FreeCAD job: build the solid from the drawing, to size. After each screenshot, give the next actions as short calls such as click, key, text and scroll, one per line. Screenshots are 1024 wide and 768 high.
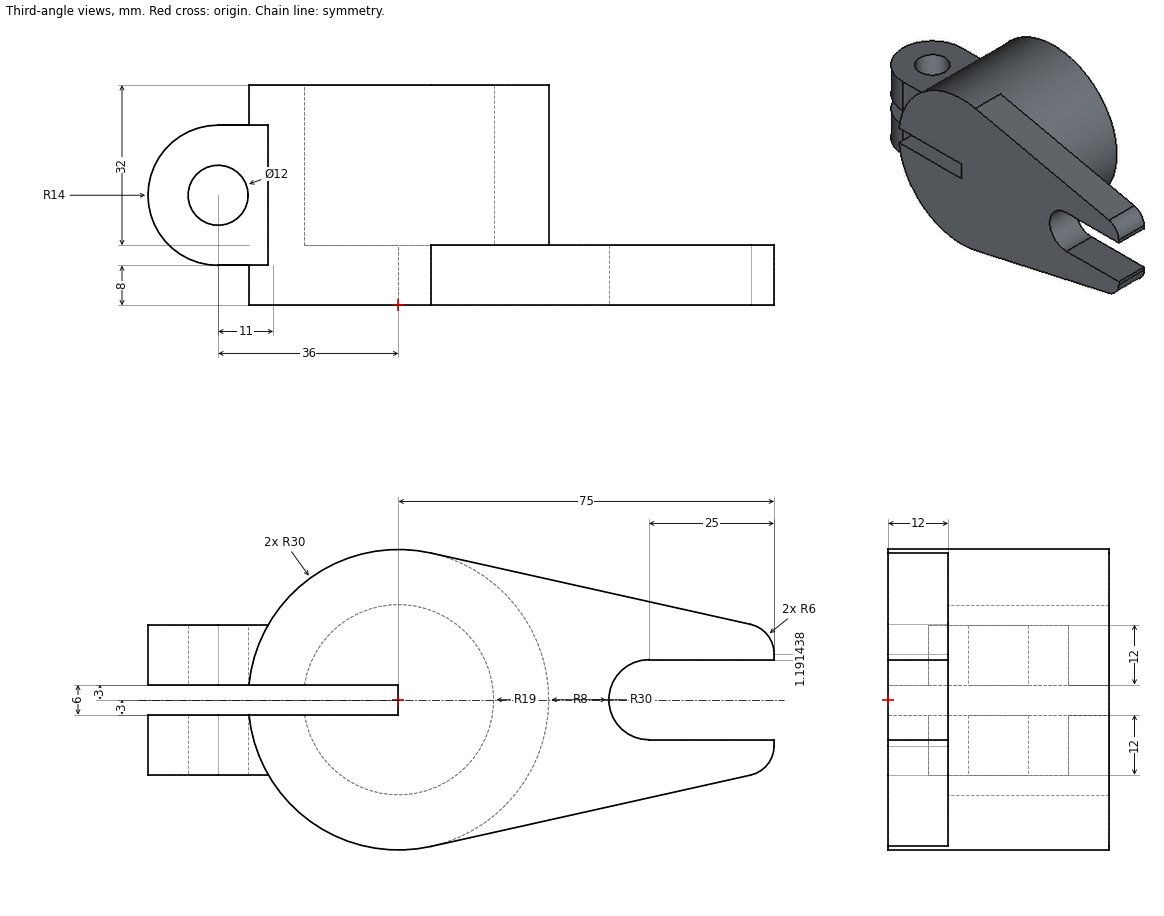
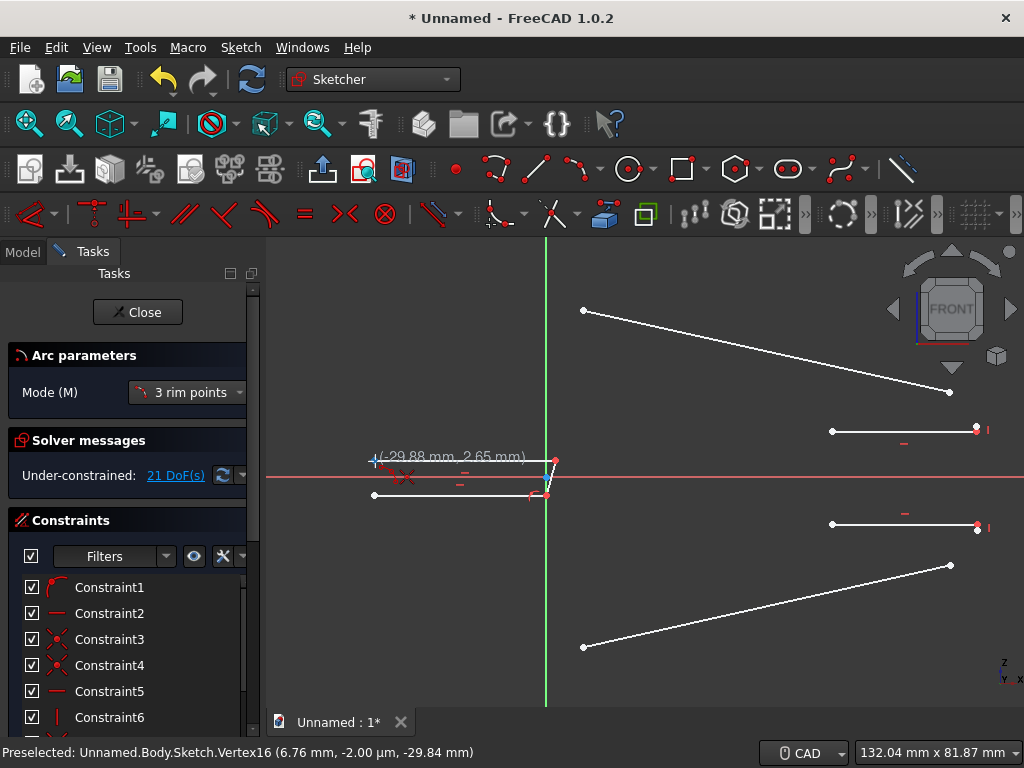
click(375, 461)
click(584, 311)
click(446, 338)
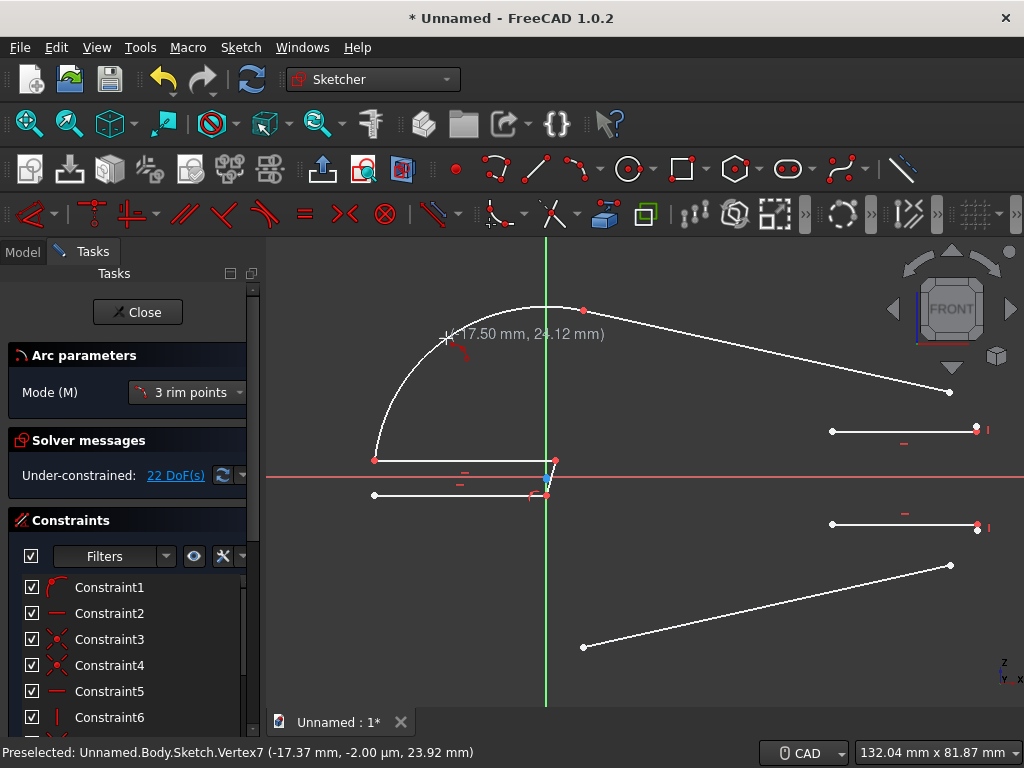
scroll(374, 461, down, 2)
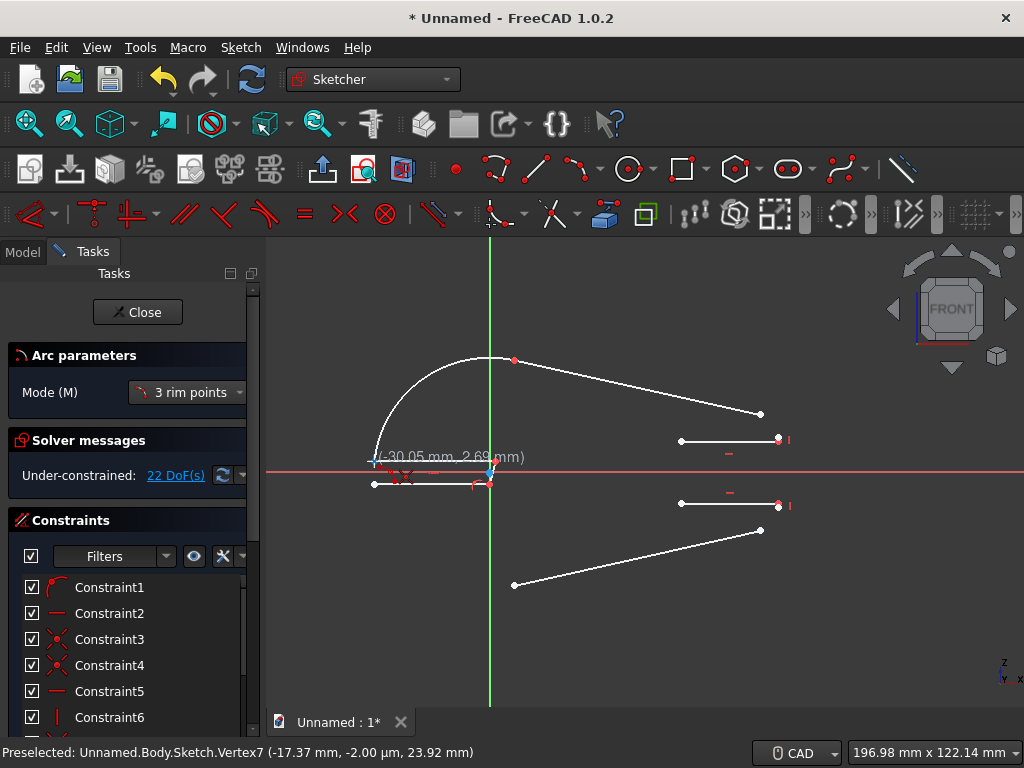
click(760, 415)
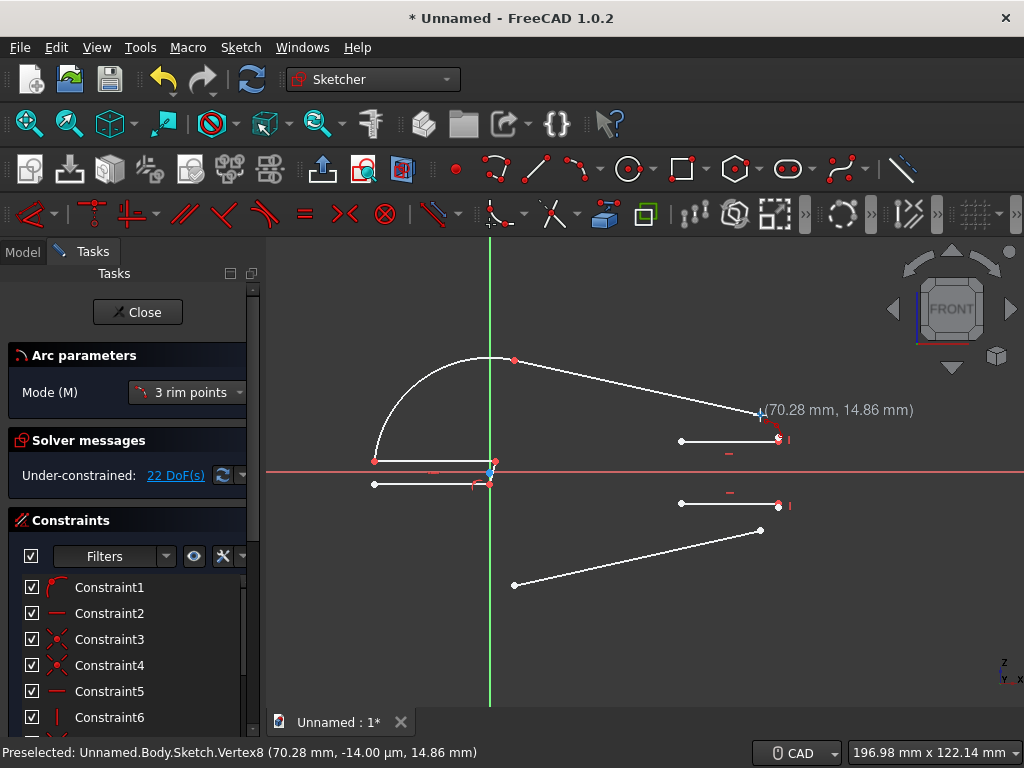
scroll(778, 437, up, 10)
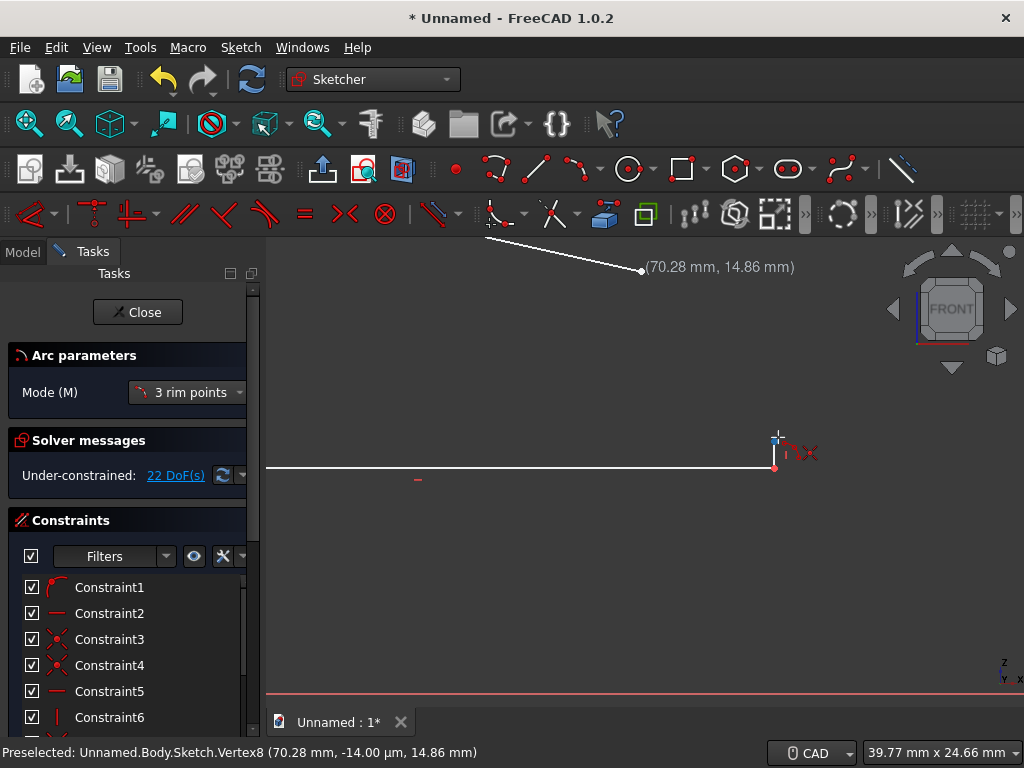
click(774, 442)
click(738, 326)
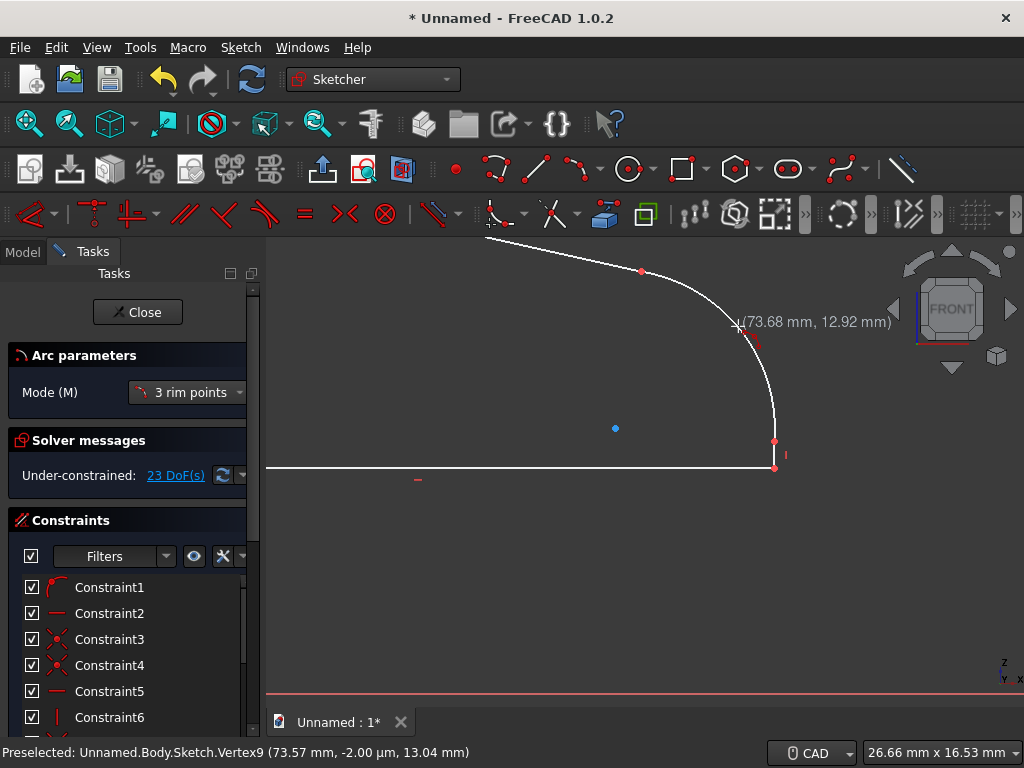
scroll(779, 437, down, 10)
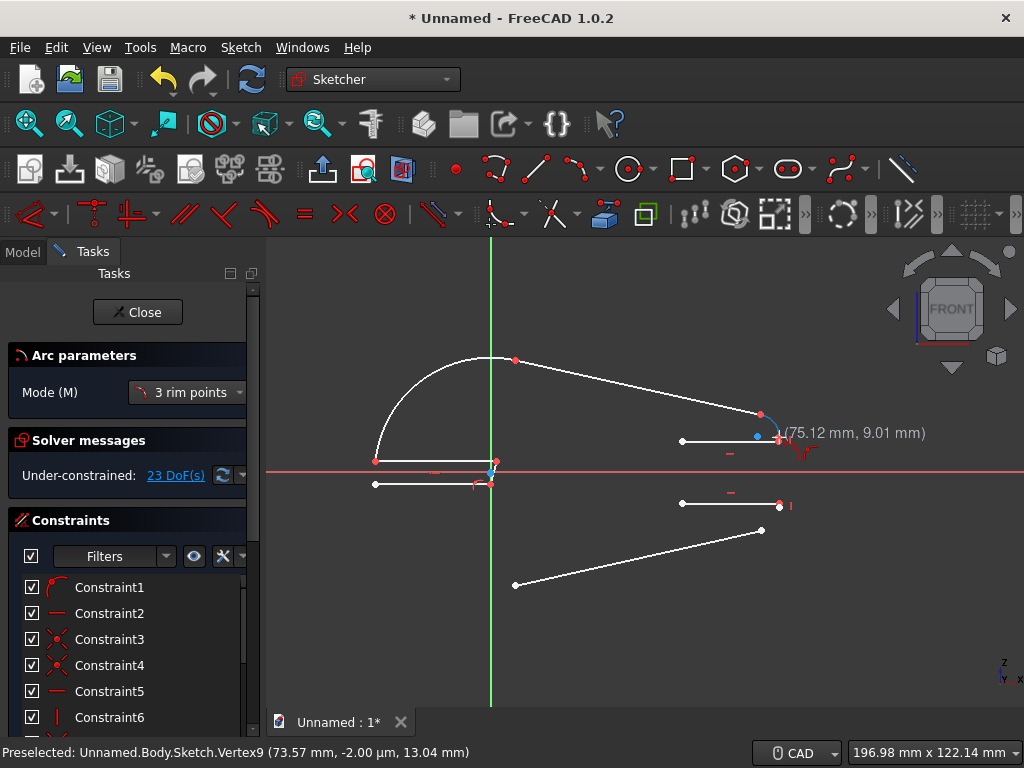
click(683, 442)
click(683, 504)
click(658, 454)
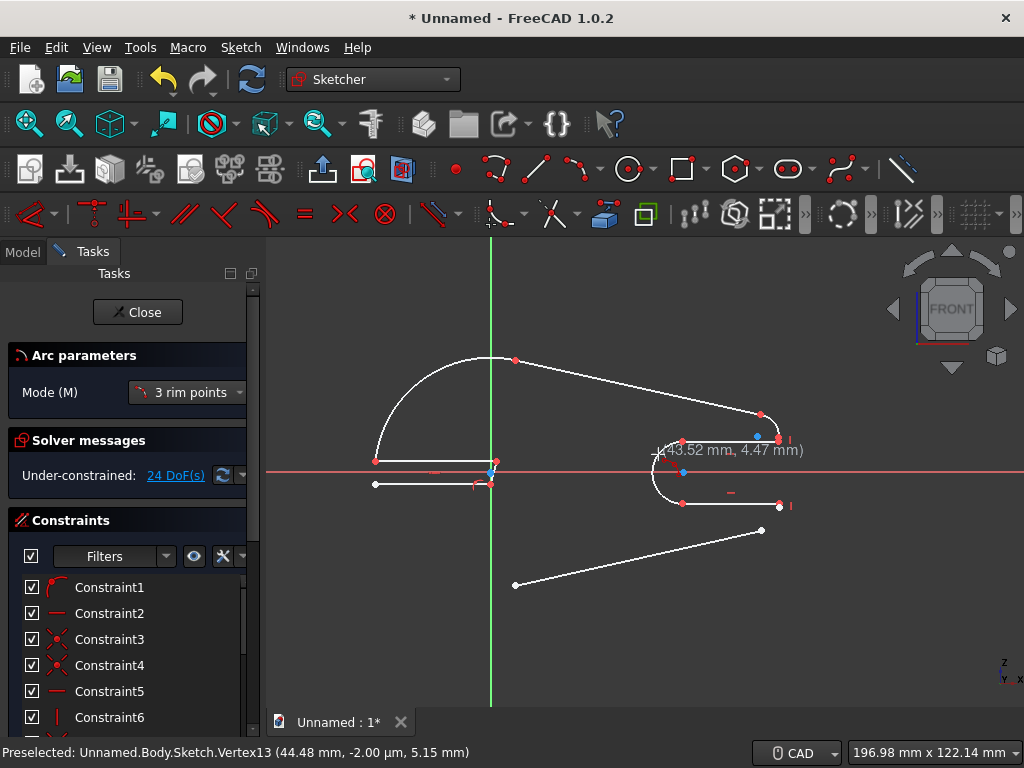
scroll(779, 508, up, 10)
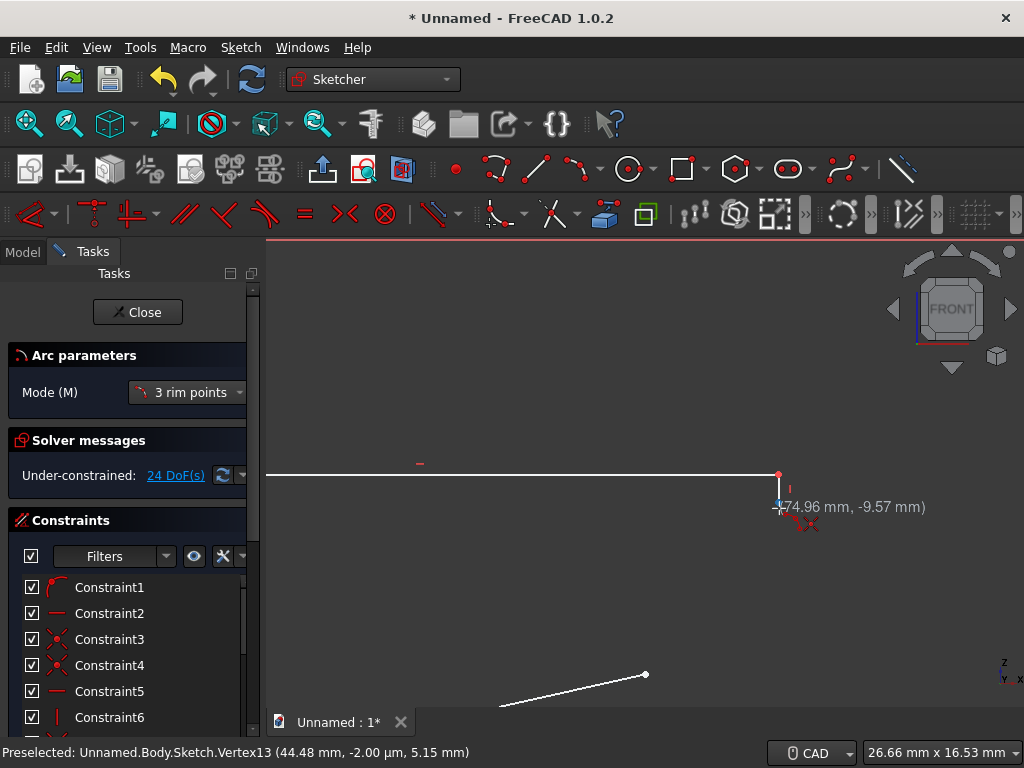
click(779, 502)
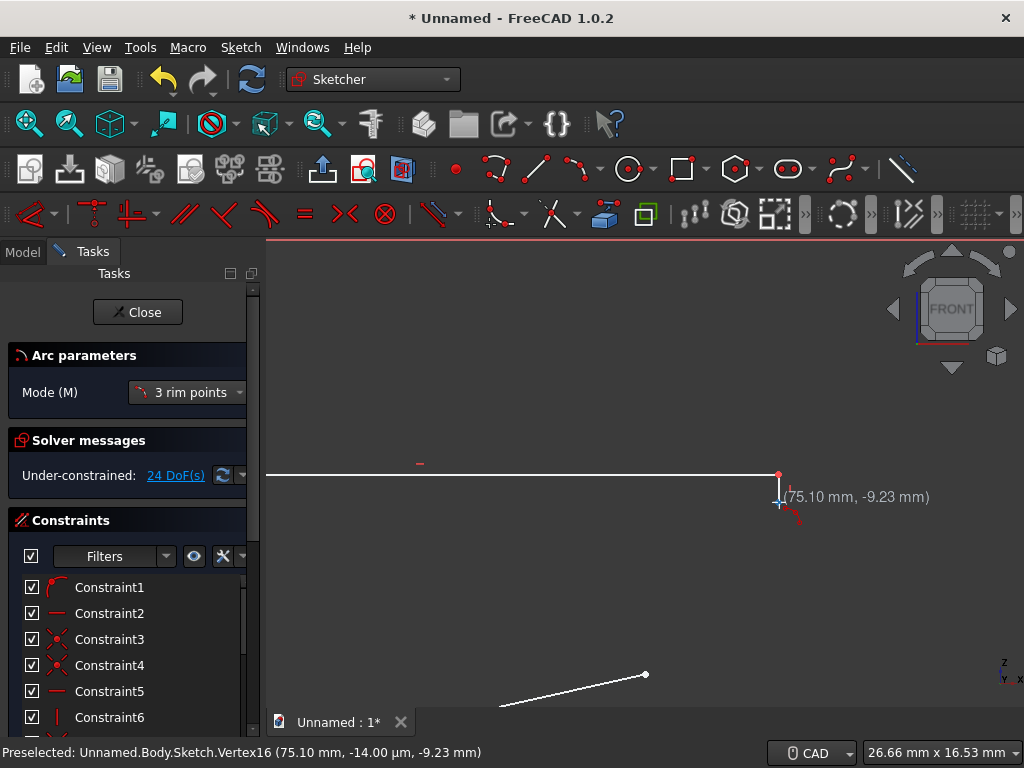
scroll(779, 508, down, 10)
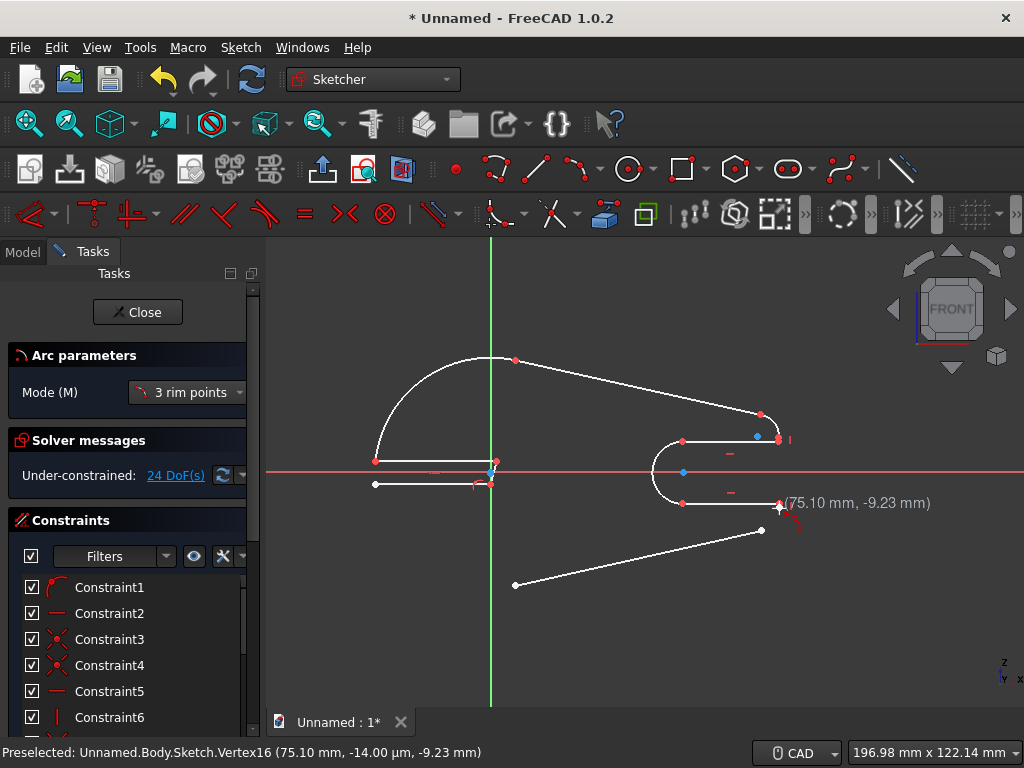
click(762, 531)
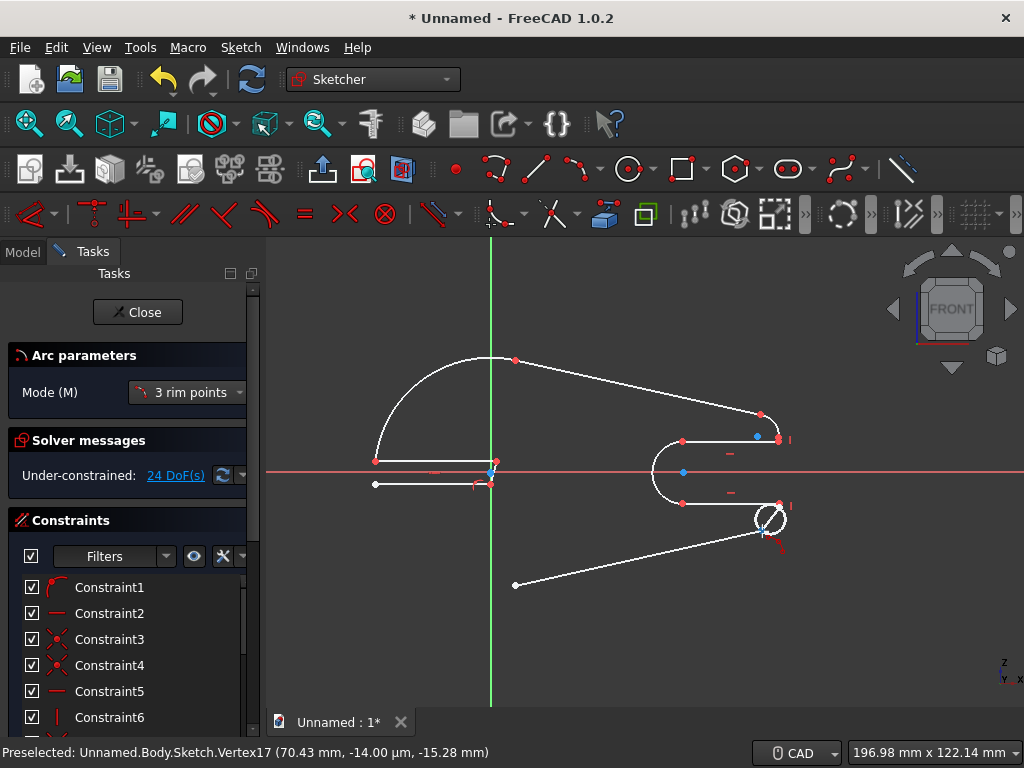
scroll(774, 522, up, 6)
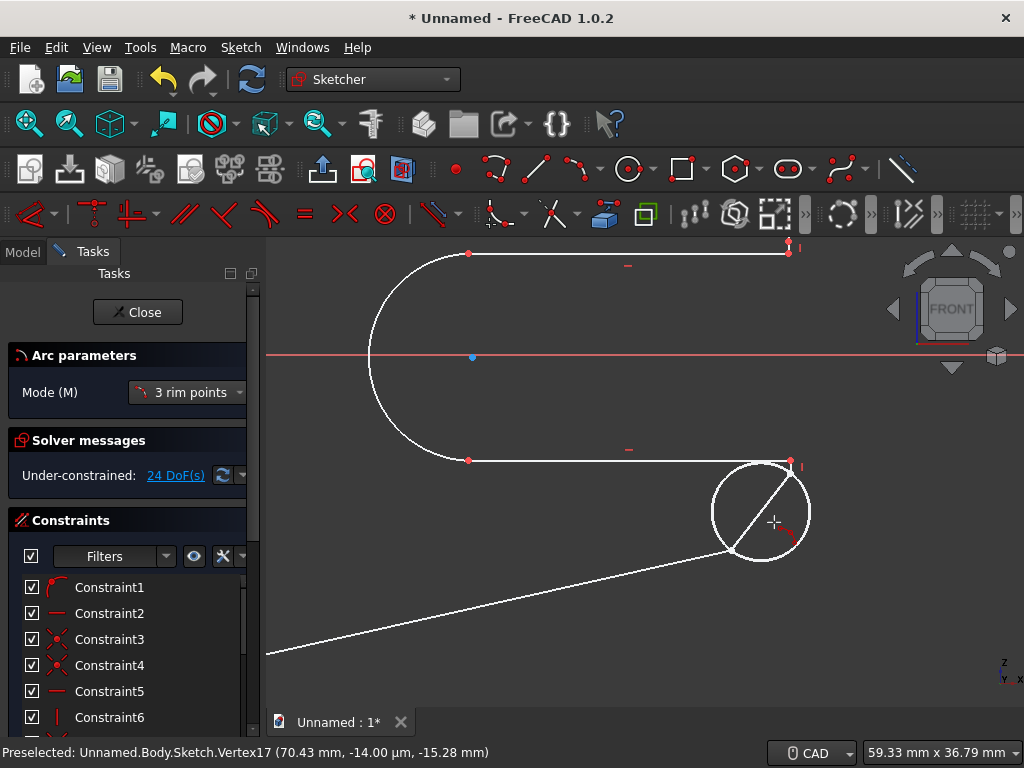
click(773, 521)